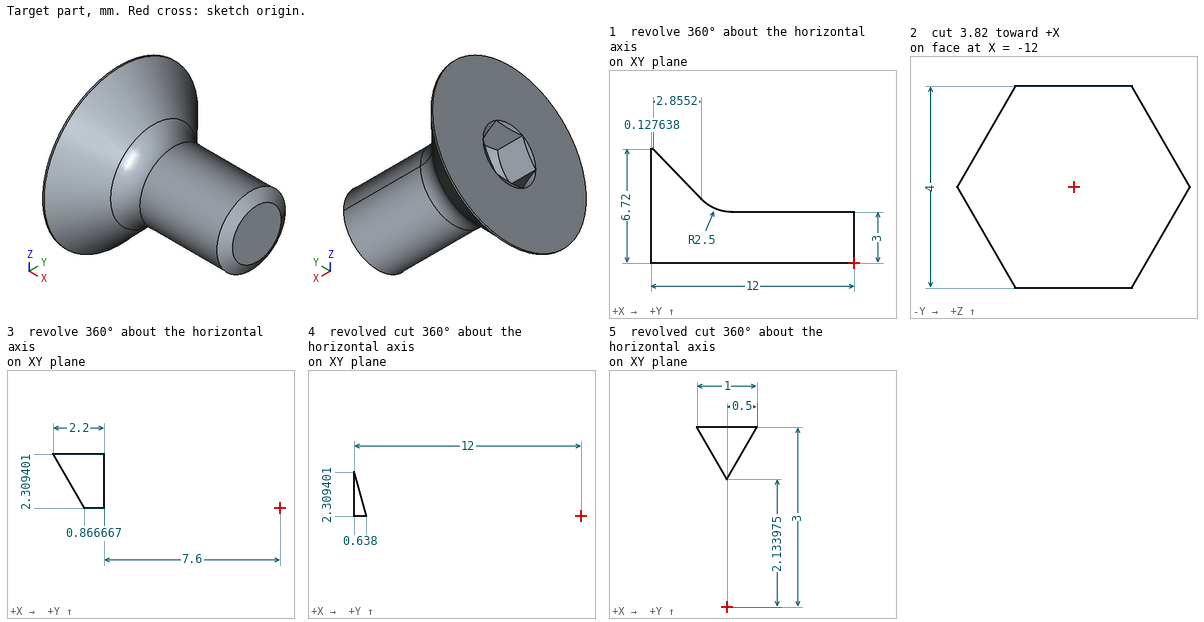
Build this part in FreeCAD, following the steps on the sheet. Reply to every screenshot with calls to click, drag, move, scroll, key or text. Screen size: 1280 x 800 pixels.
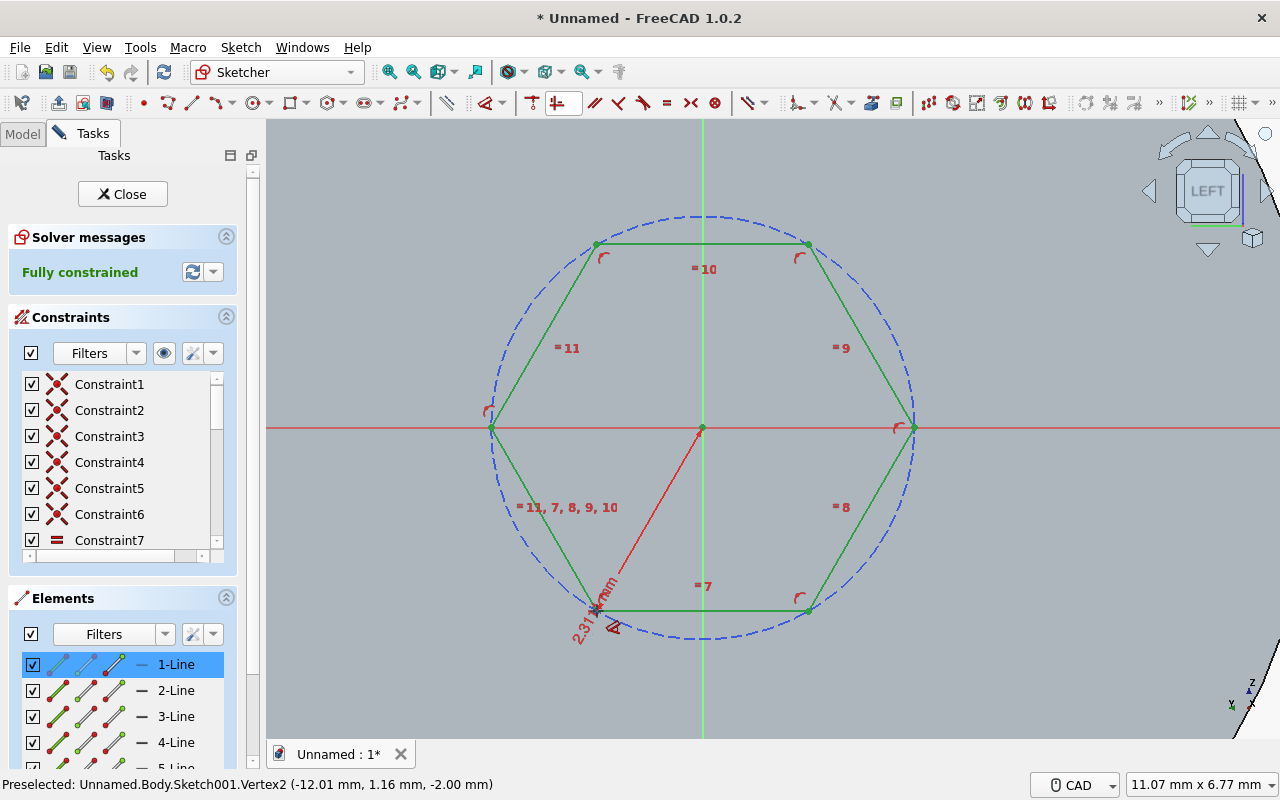
click(809, 244)
click(843, 343)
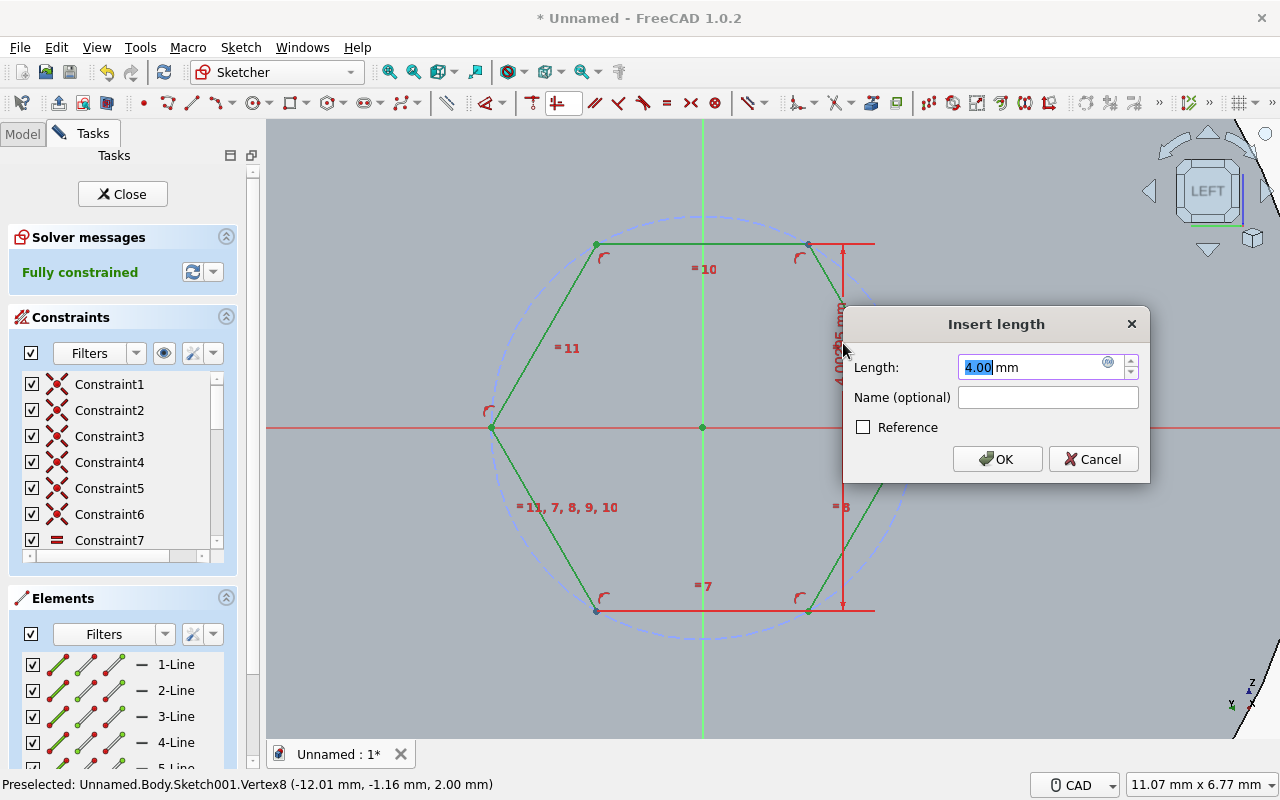
text(4)
key(Return)
key(Escape)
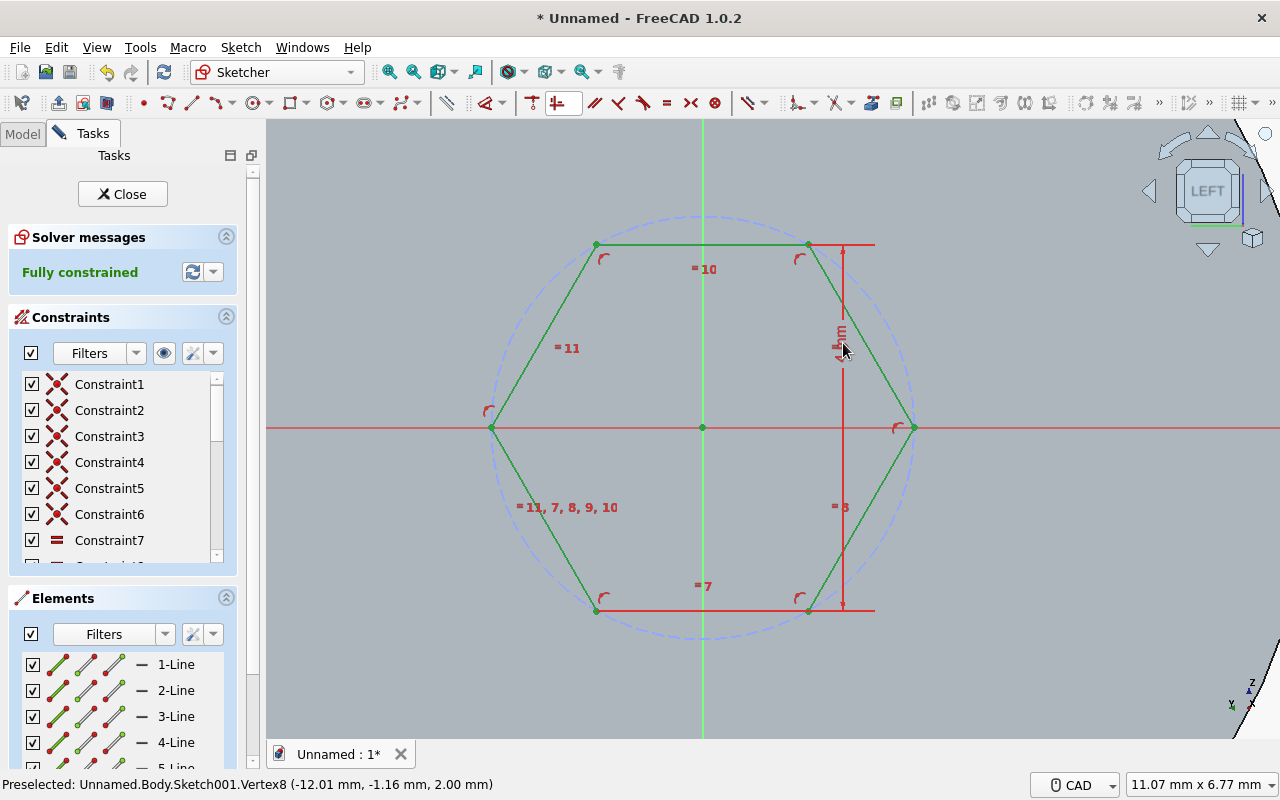
click(123, 194)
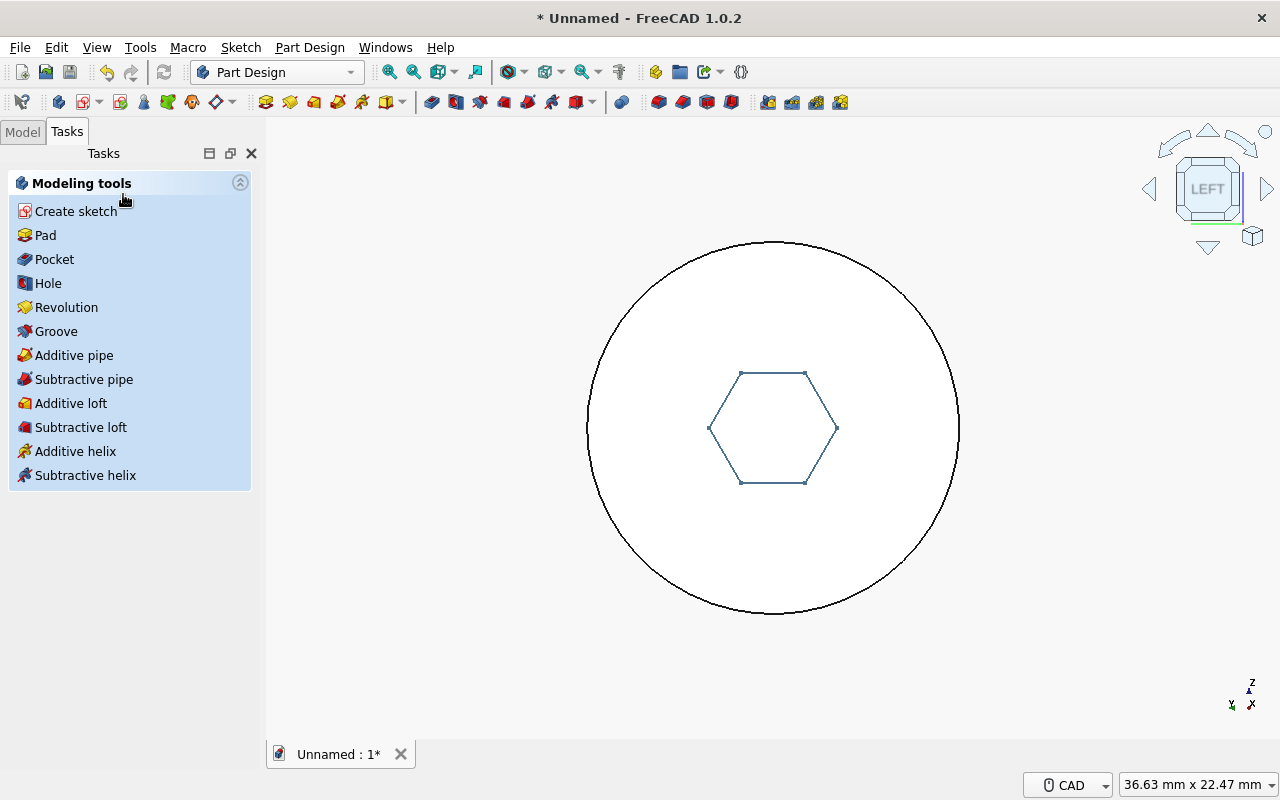
click(432, 102)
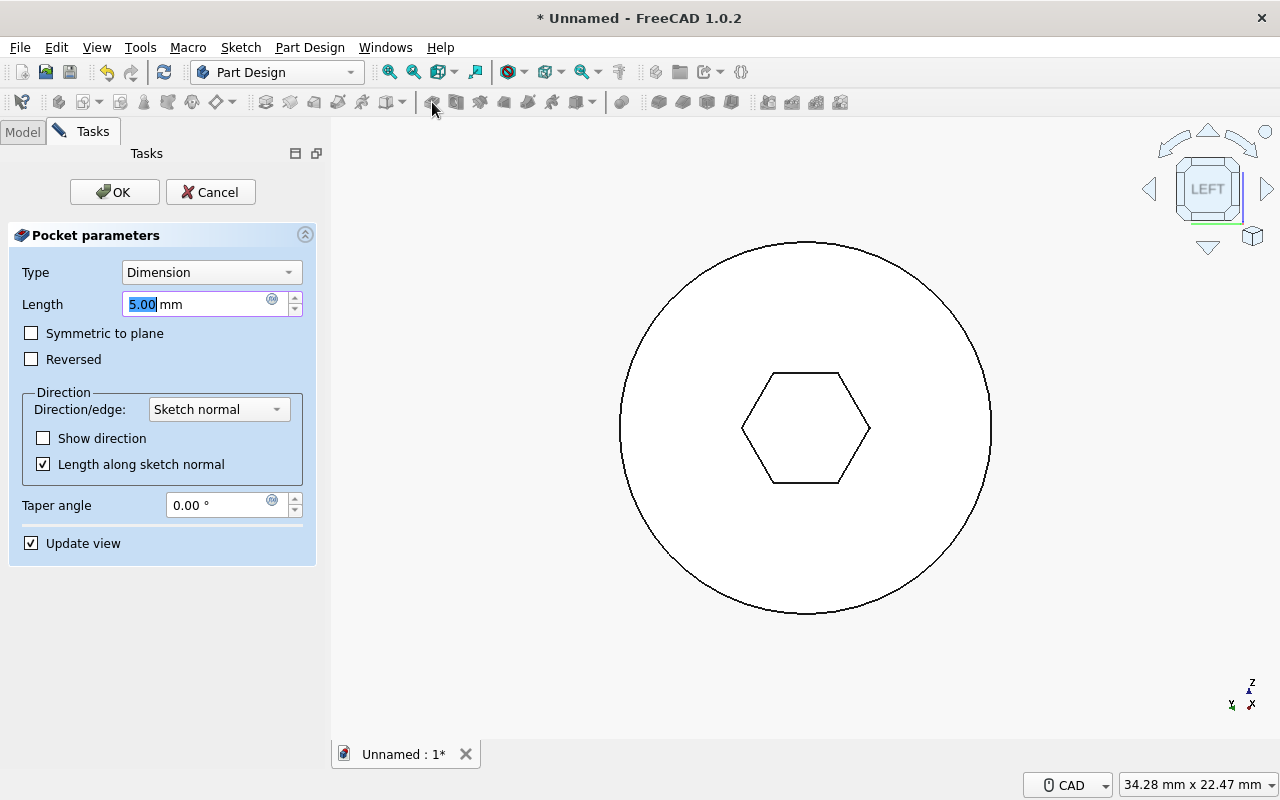
text(3.82)
key(Tab)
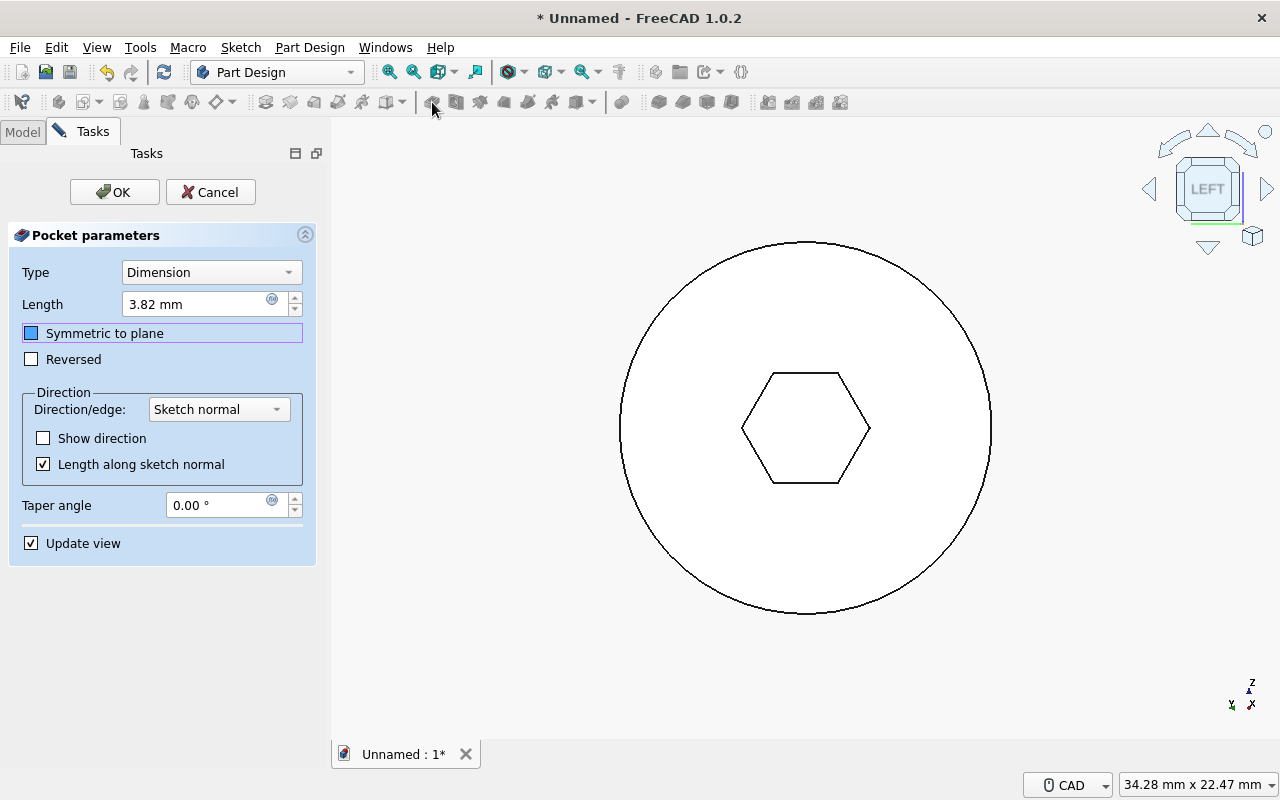
click(115, 192)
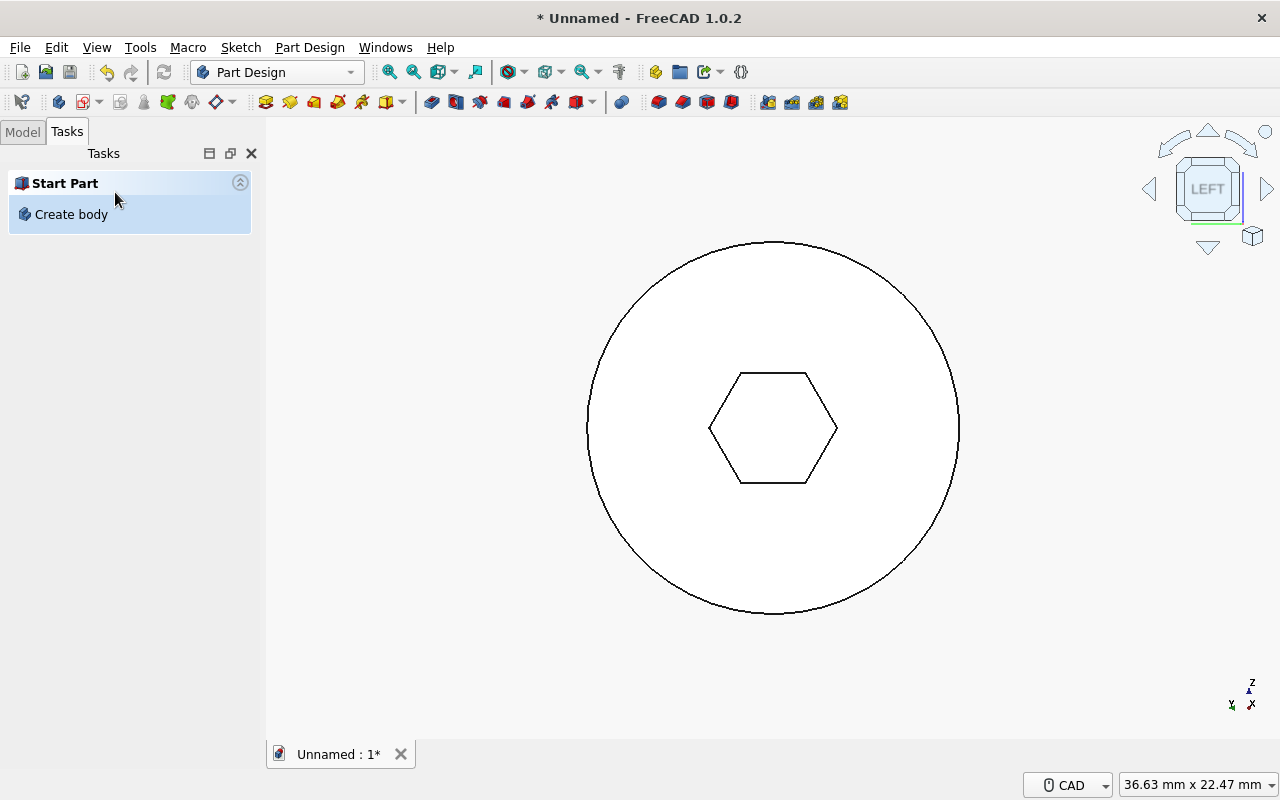
click(84, 102)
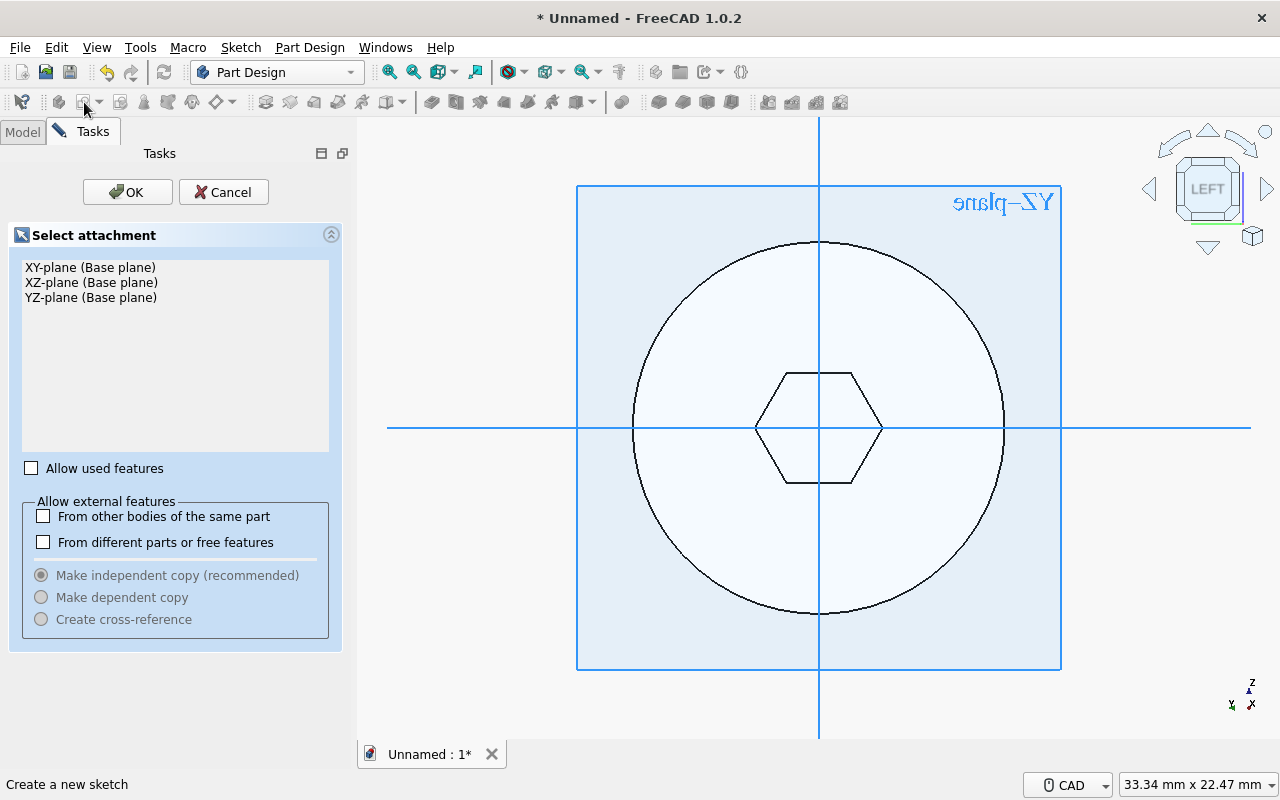
click(82, 268)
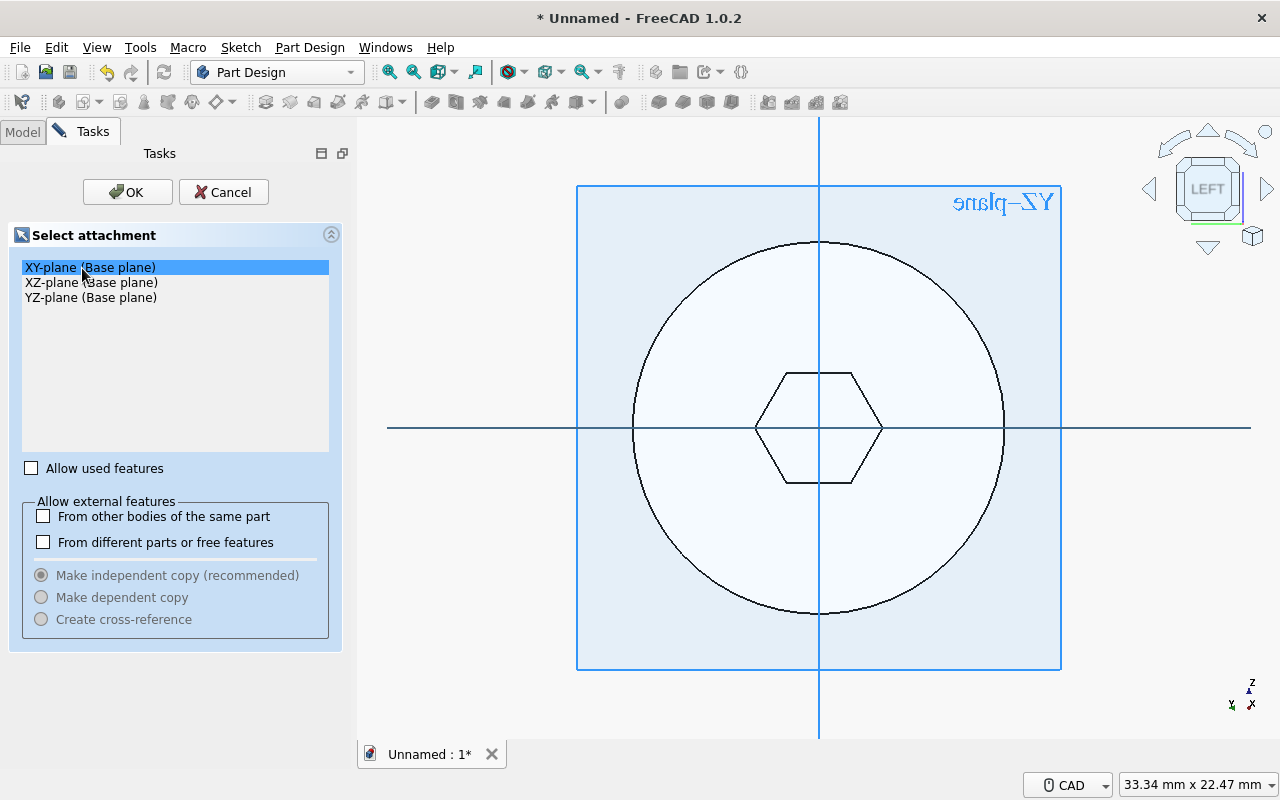
click(128, 192)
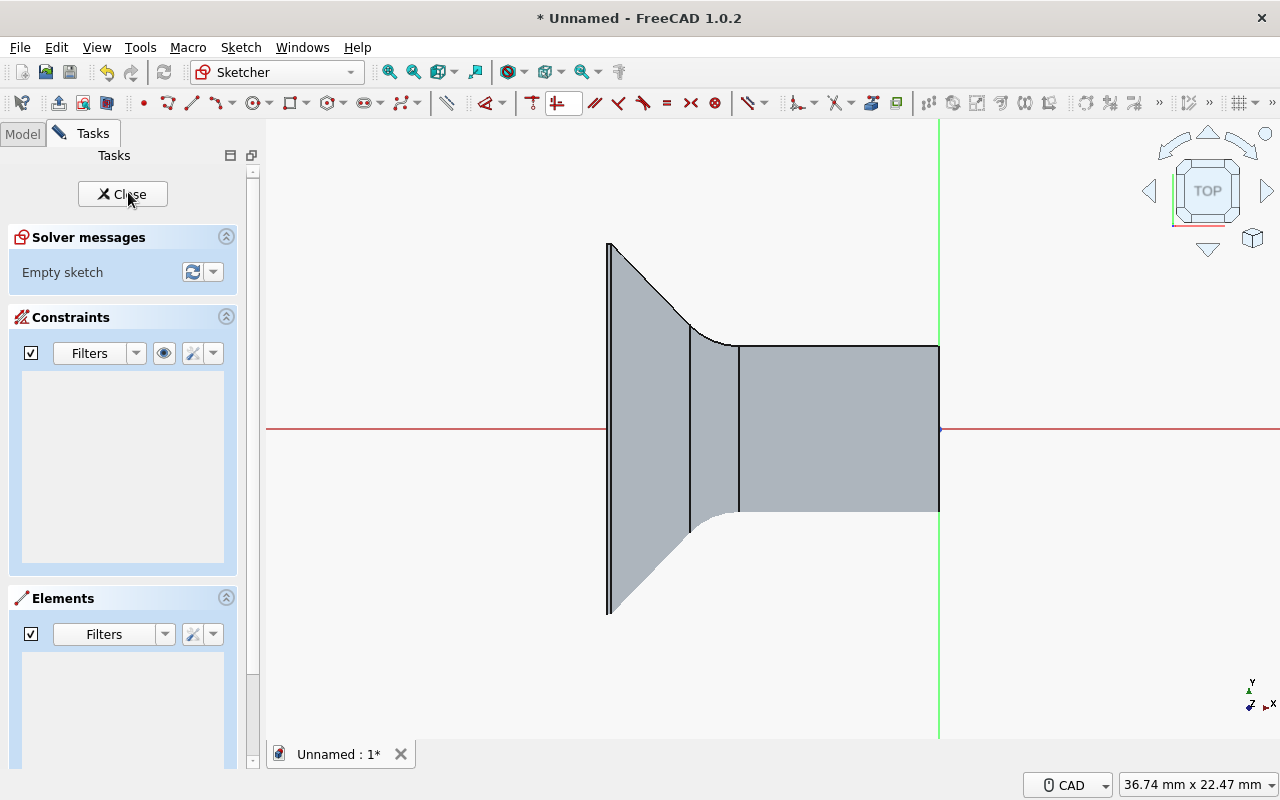
key(q)
key(s)